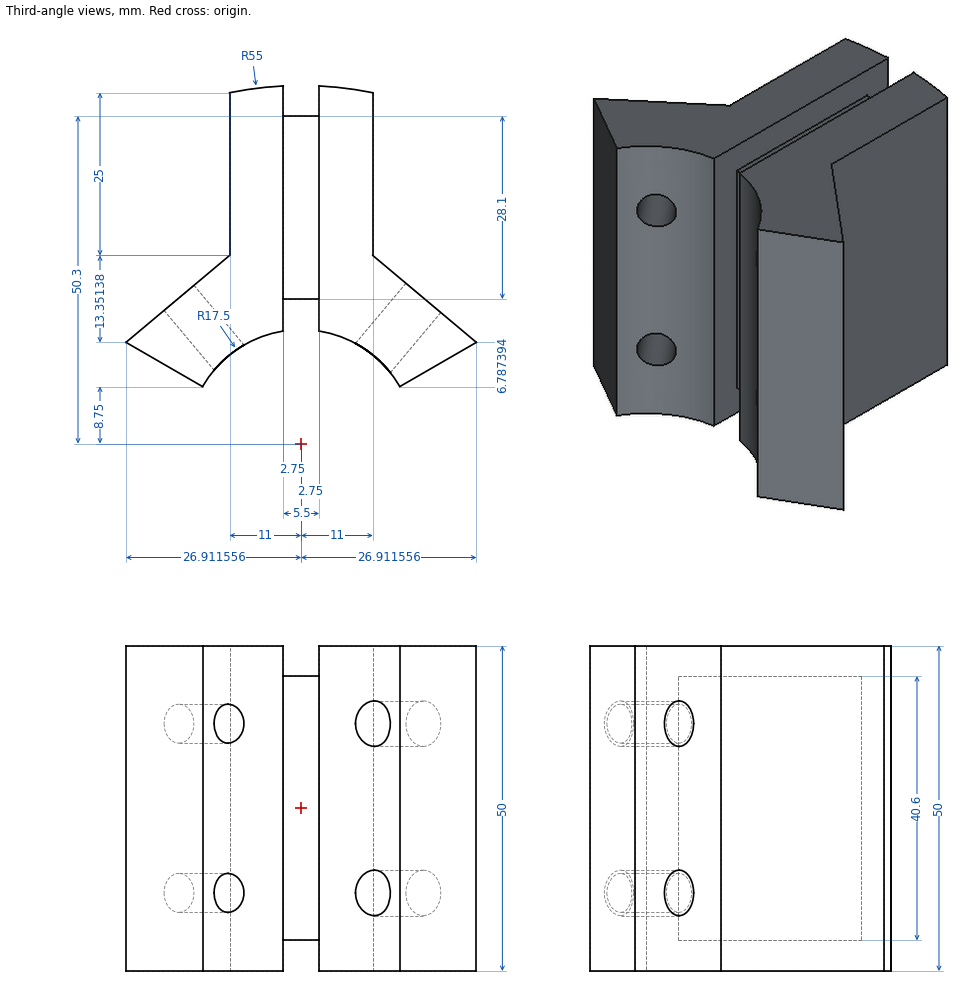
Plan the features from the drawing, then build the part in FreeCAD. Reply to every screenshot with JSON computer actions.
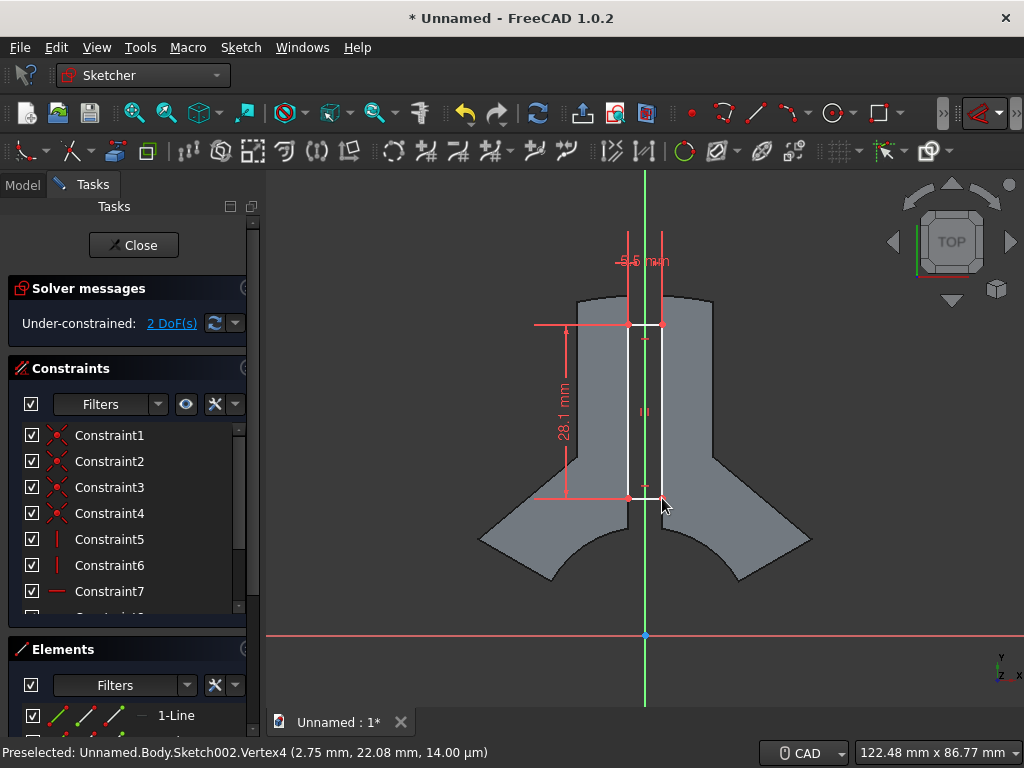
{"action": "scroll", "coordinate": [628, 325], "scroll_direction": "up", "scroll_amount": 5}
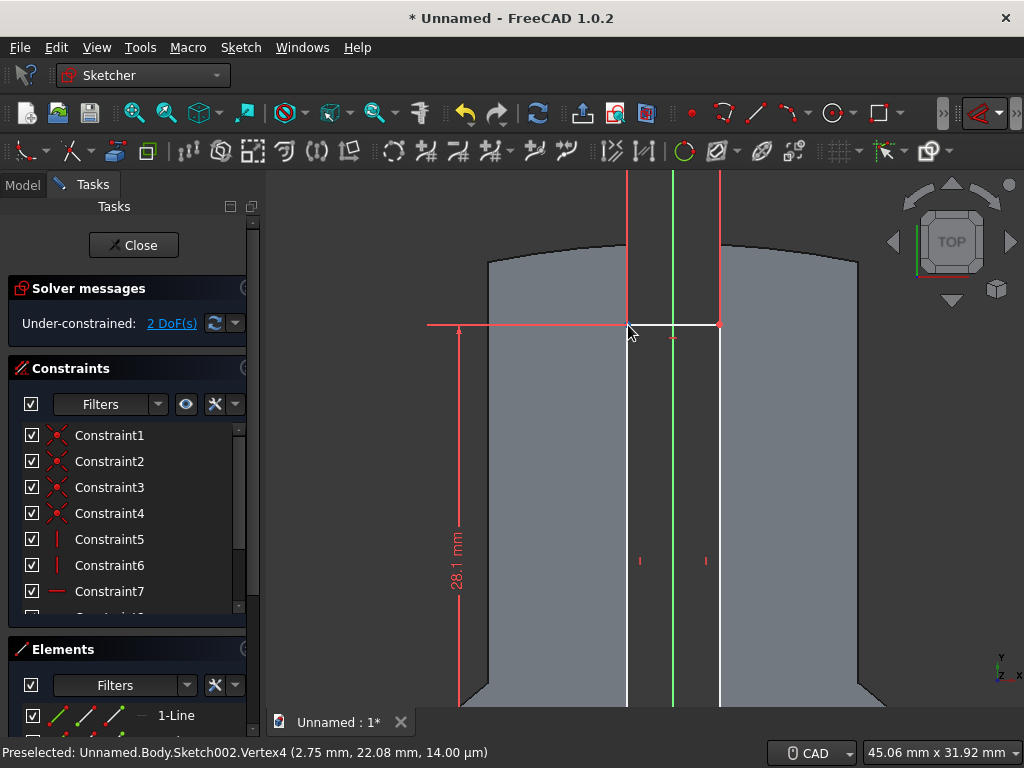
{"action": "left_click", "coordinate": [627, 325]}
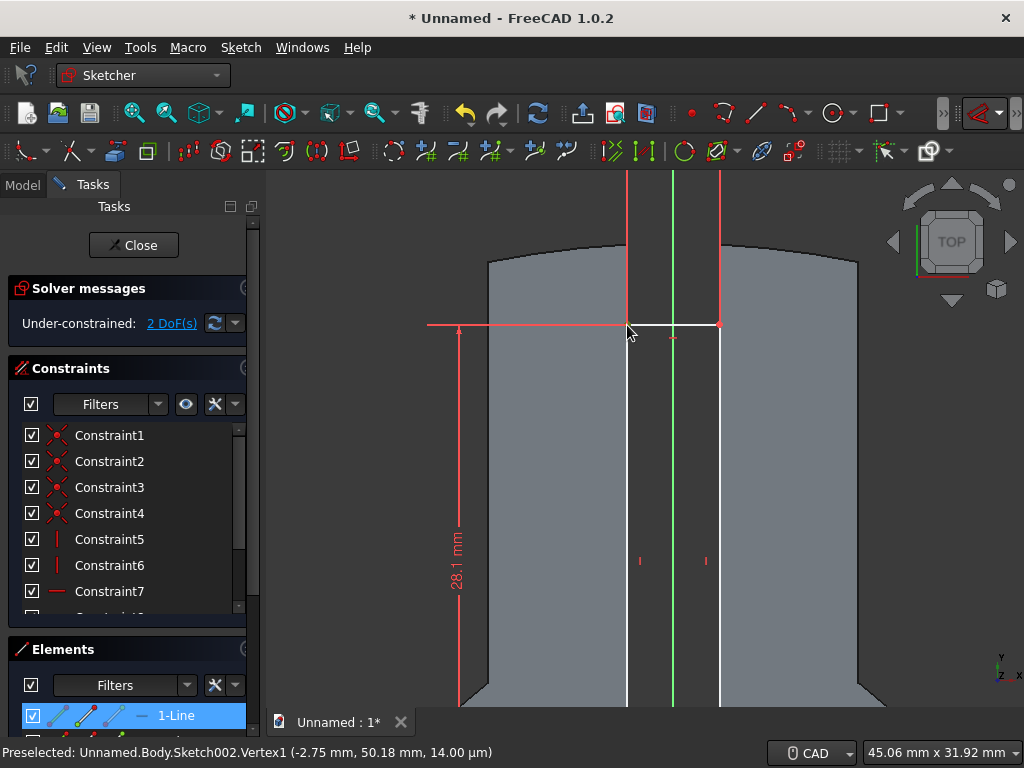
{"action": "left_click", "coordinate": [1002, 114]}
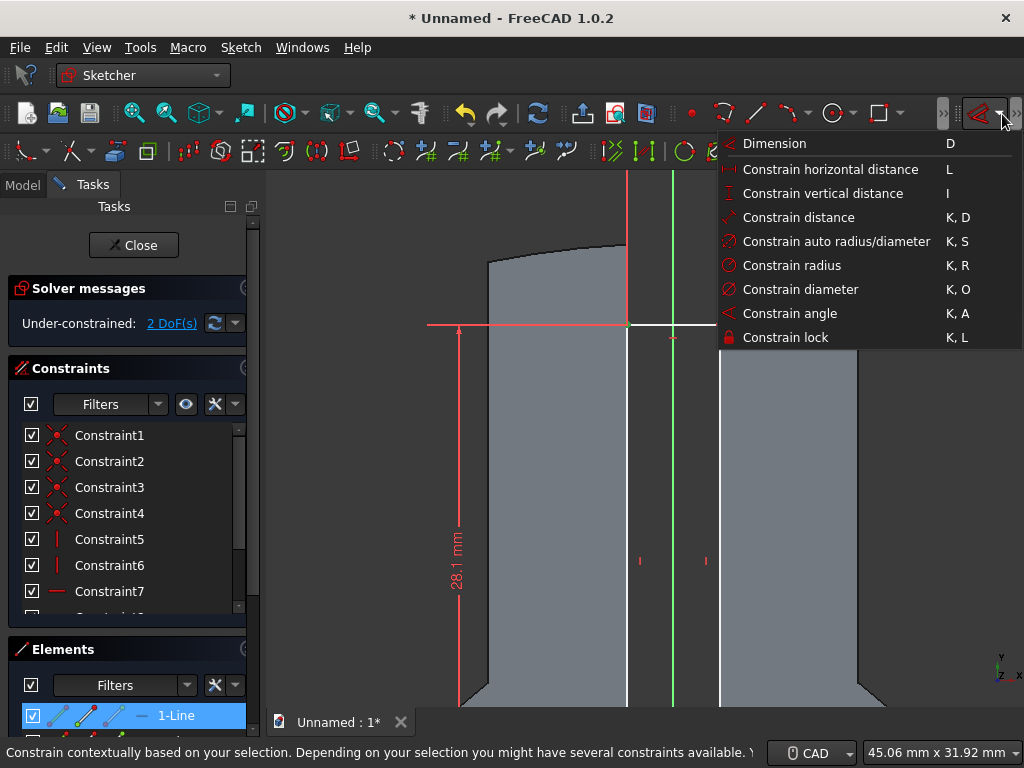
{"action": "left_click", "coordinate": [870, 169]}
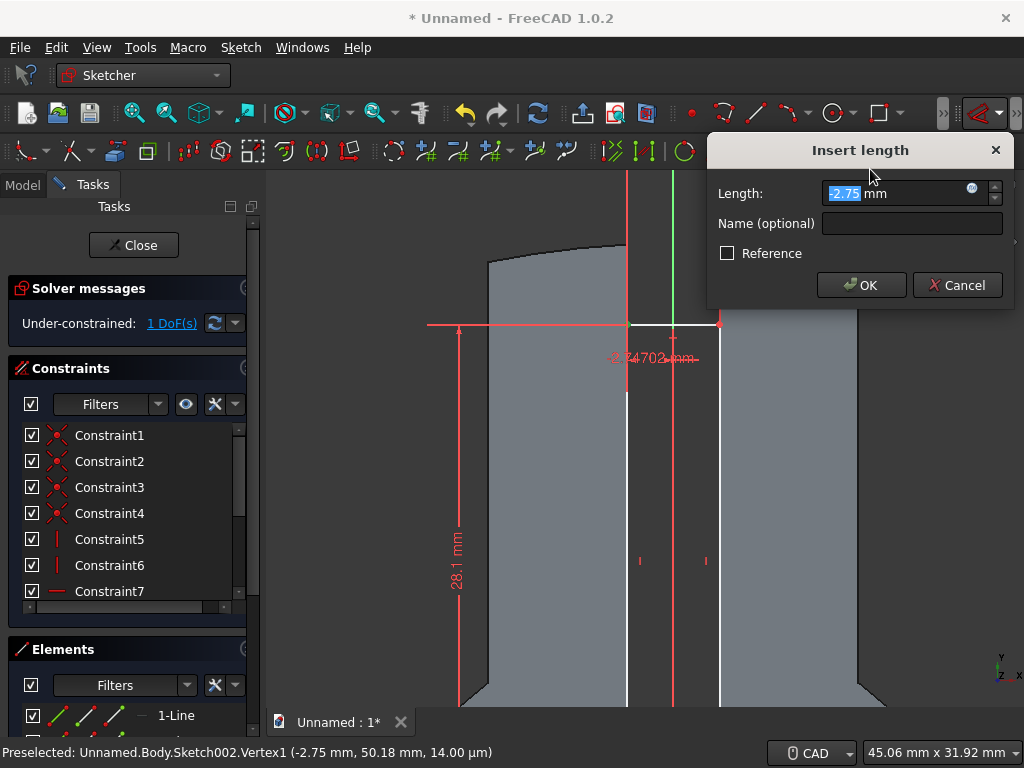
{"action": "type", "text": "-2.75"}
{"action": "key", "text": "Return"}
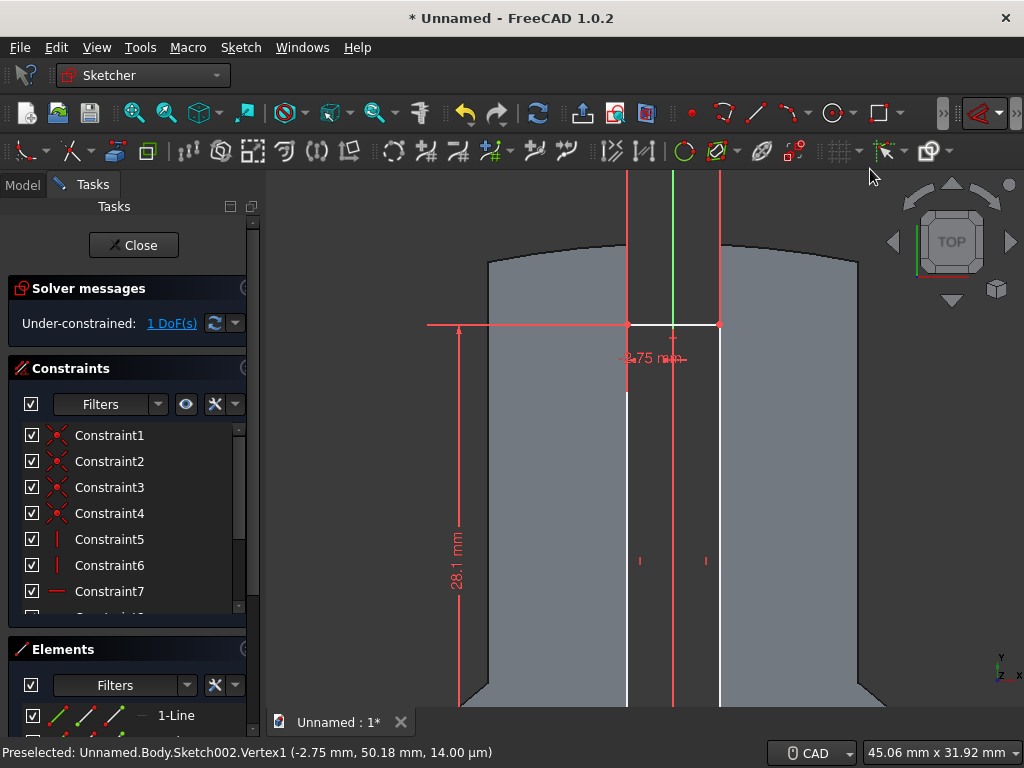
{"action": "left_click", "coordinate": [627, 325]}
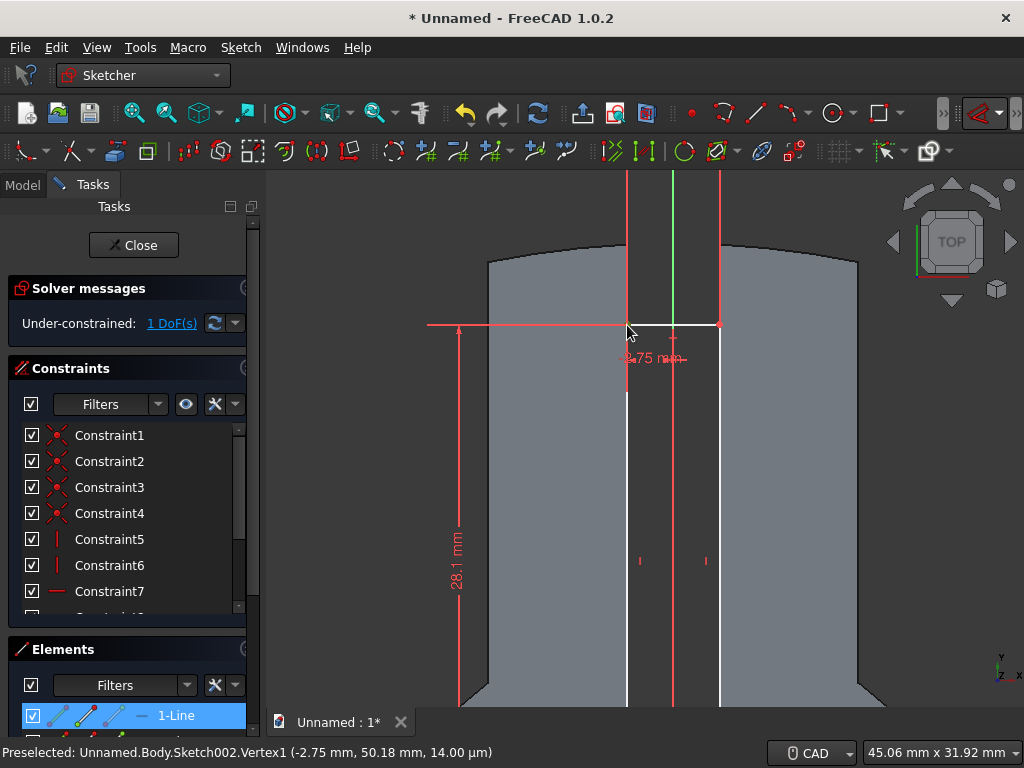
{"action": "left_click", "coordinate": [1002, 114]}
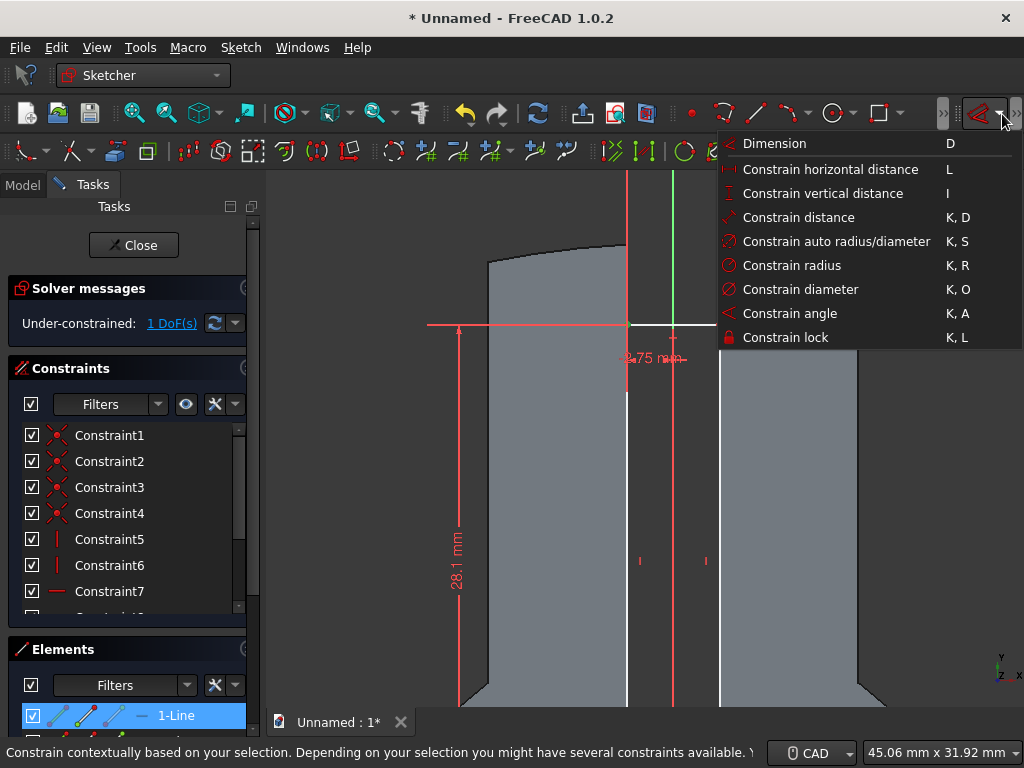
{"action": "left_click", "coordinate": [870, 193]}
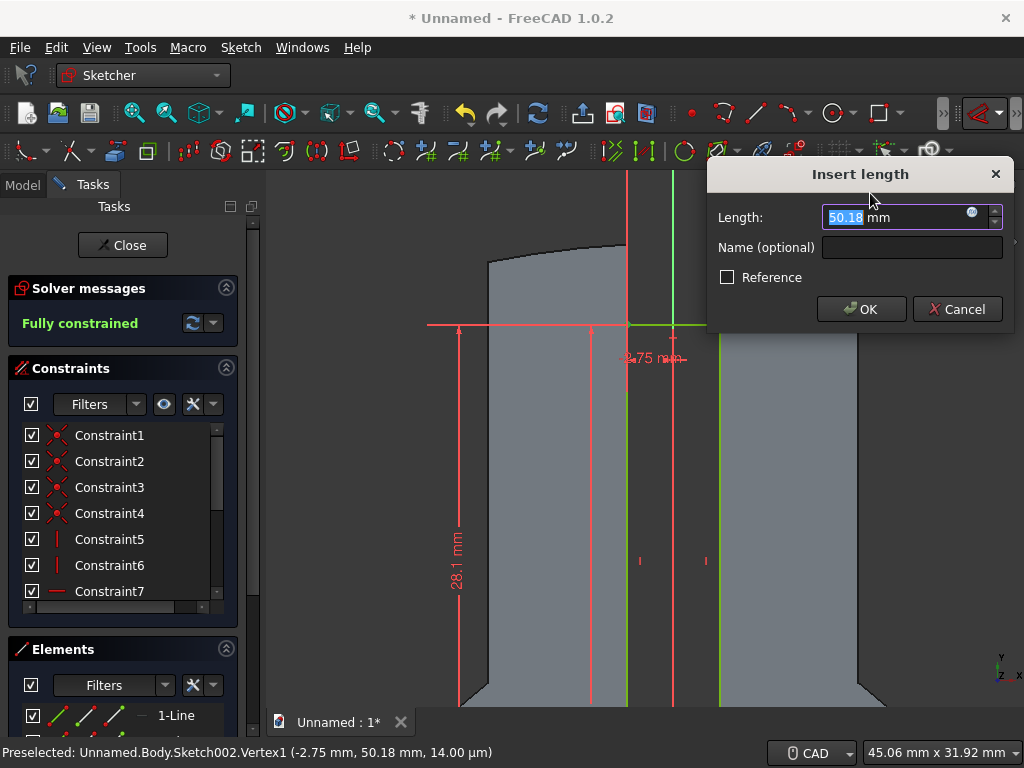
{"action": "type", "text": "50.3"}
{"action": "key", "text": "Return"}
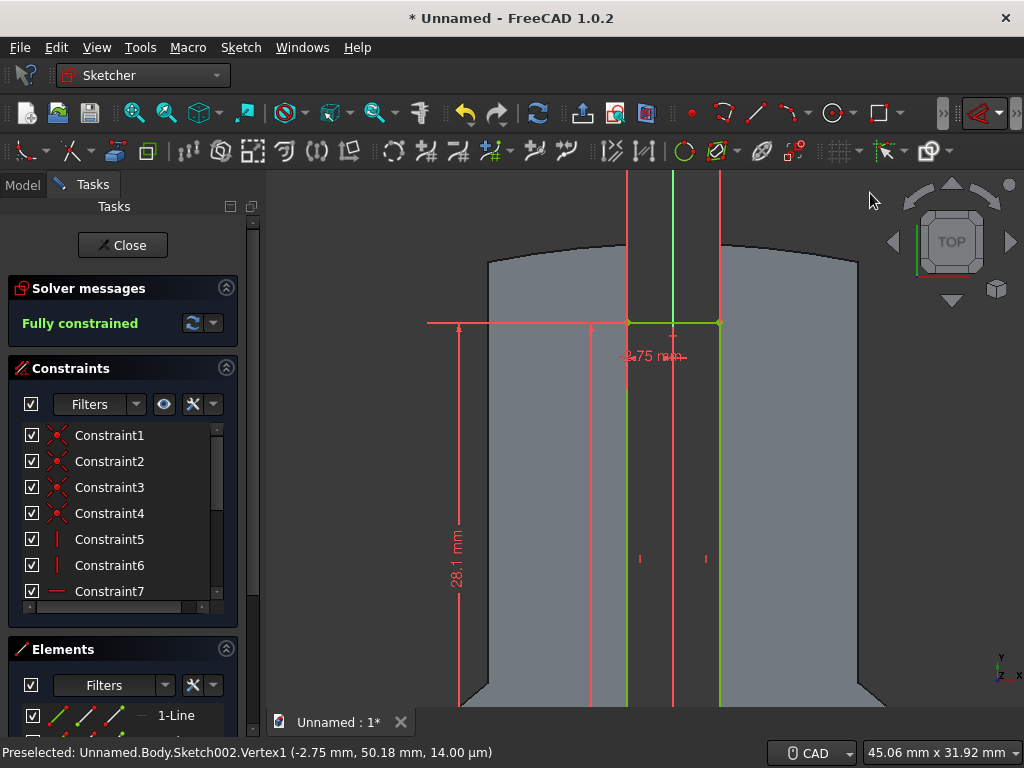
{"action": "left_click", "coordinate": [123, 245]}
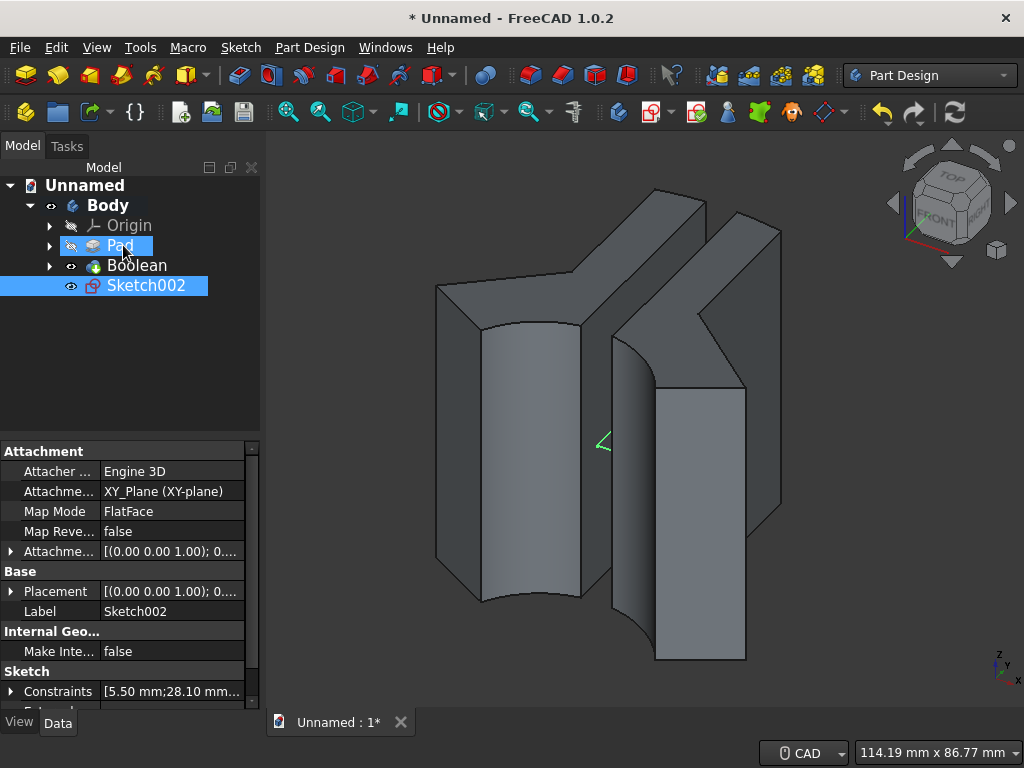
{"action": "left_click", "coordinate": [26, 76]}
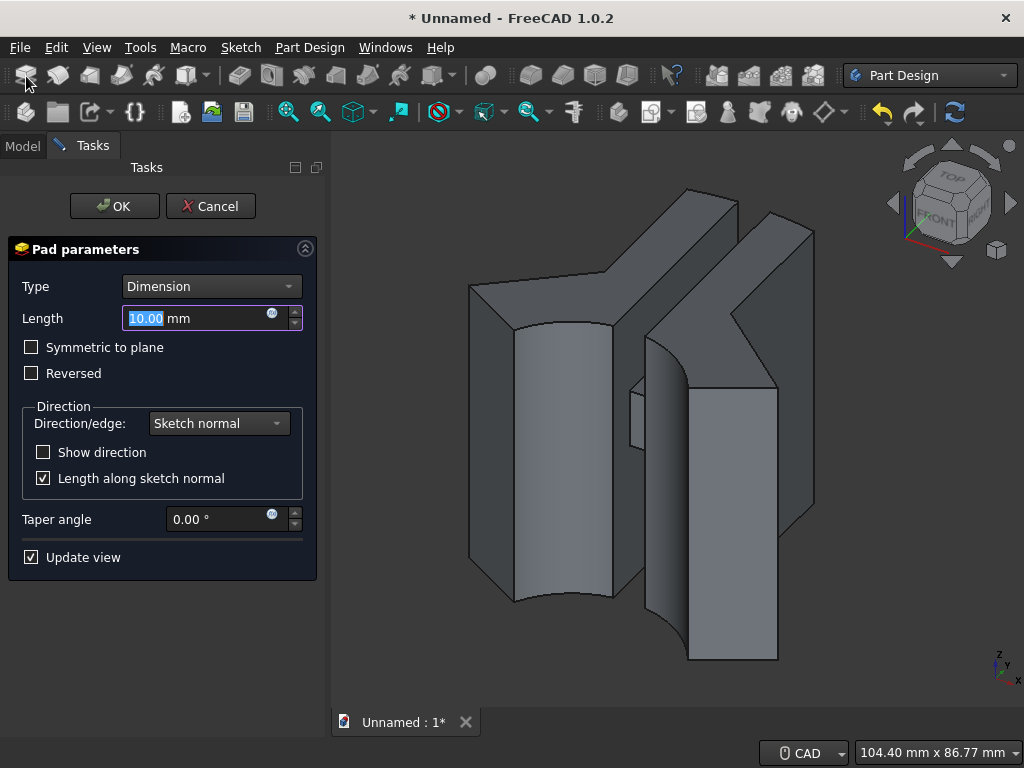
{"action": "type", "text": "40.6"}
{"action": "key", "text": "Tab"}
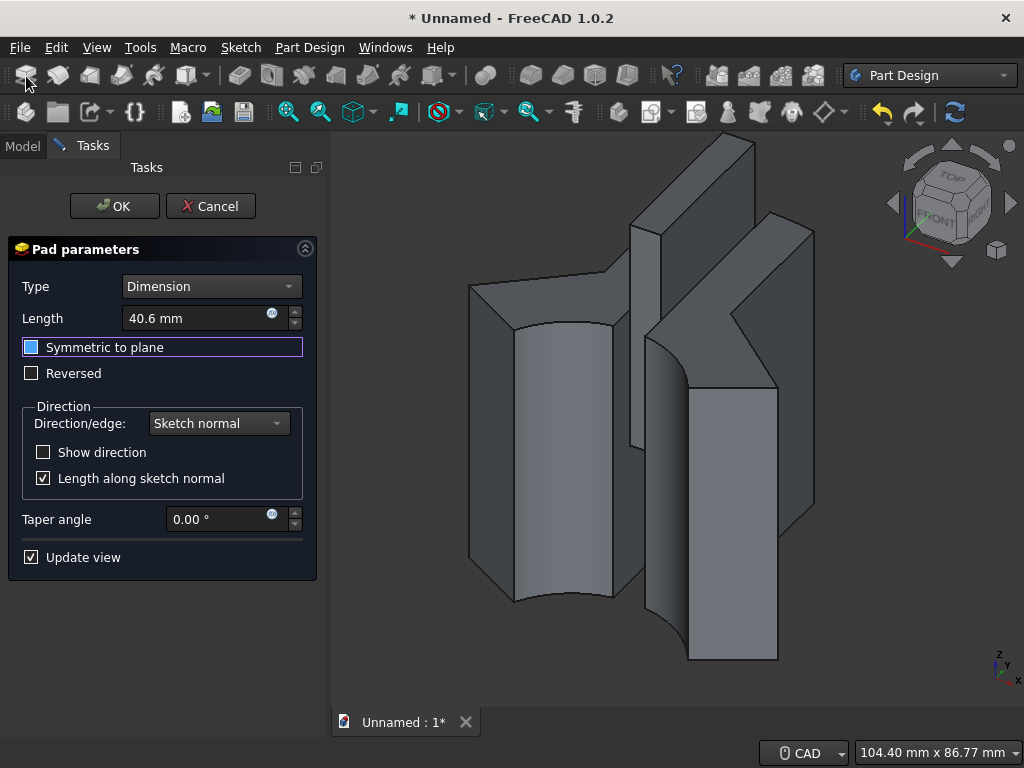
{"action": "left_click", "coordinate": [30, 347]}